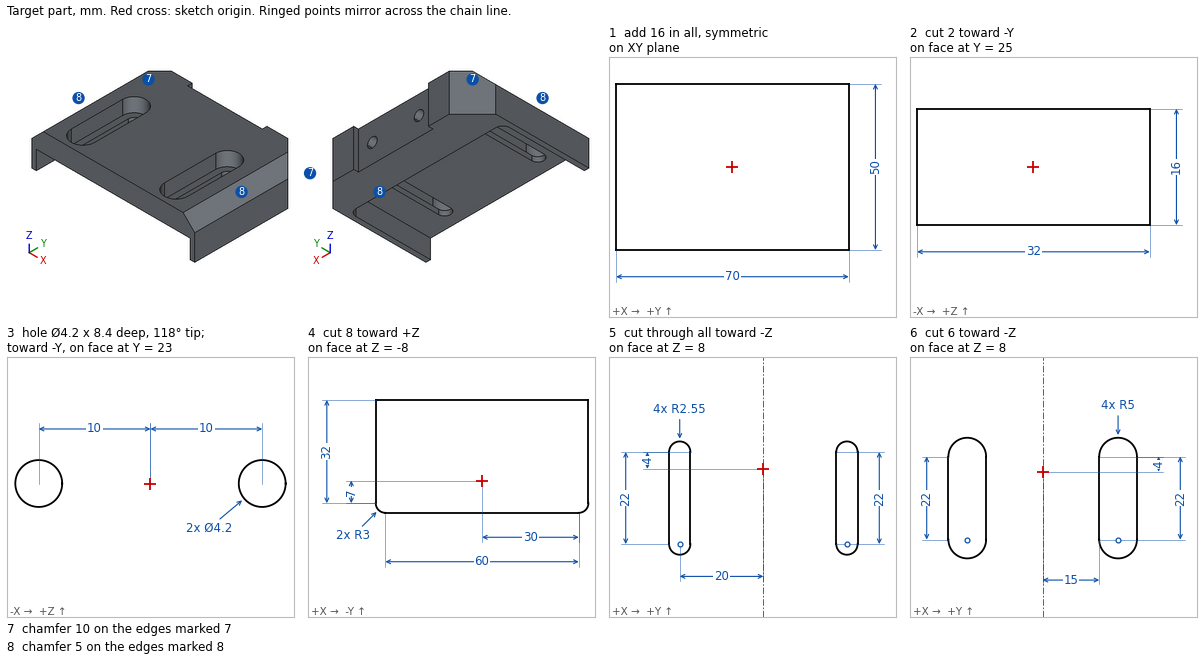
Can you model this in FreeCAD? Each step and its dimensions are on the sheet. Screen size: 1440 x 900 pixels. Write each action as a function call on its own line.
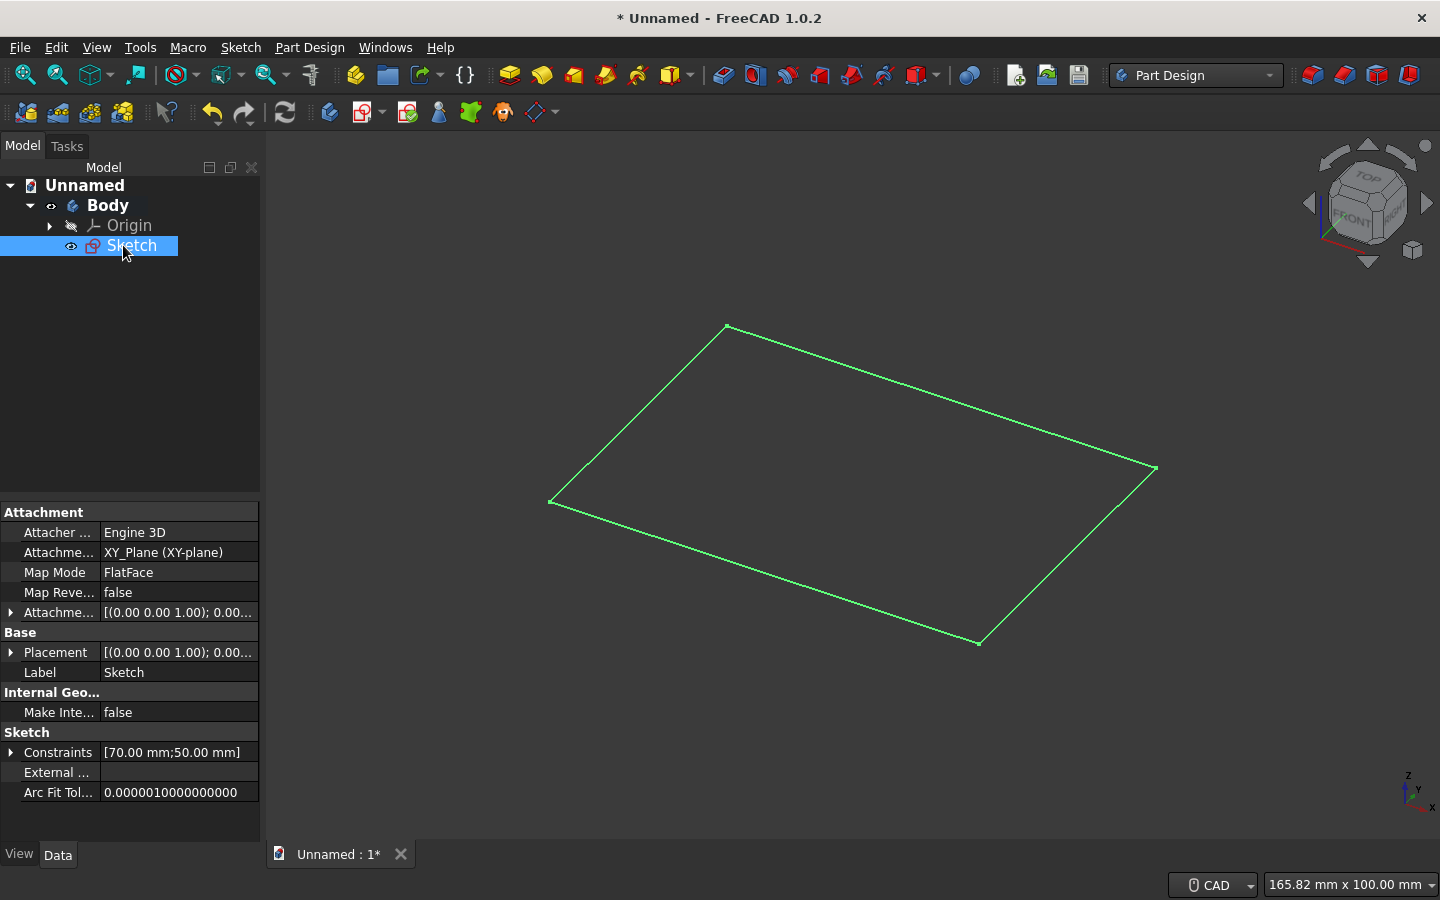
click(510, 76)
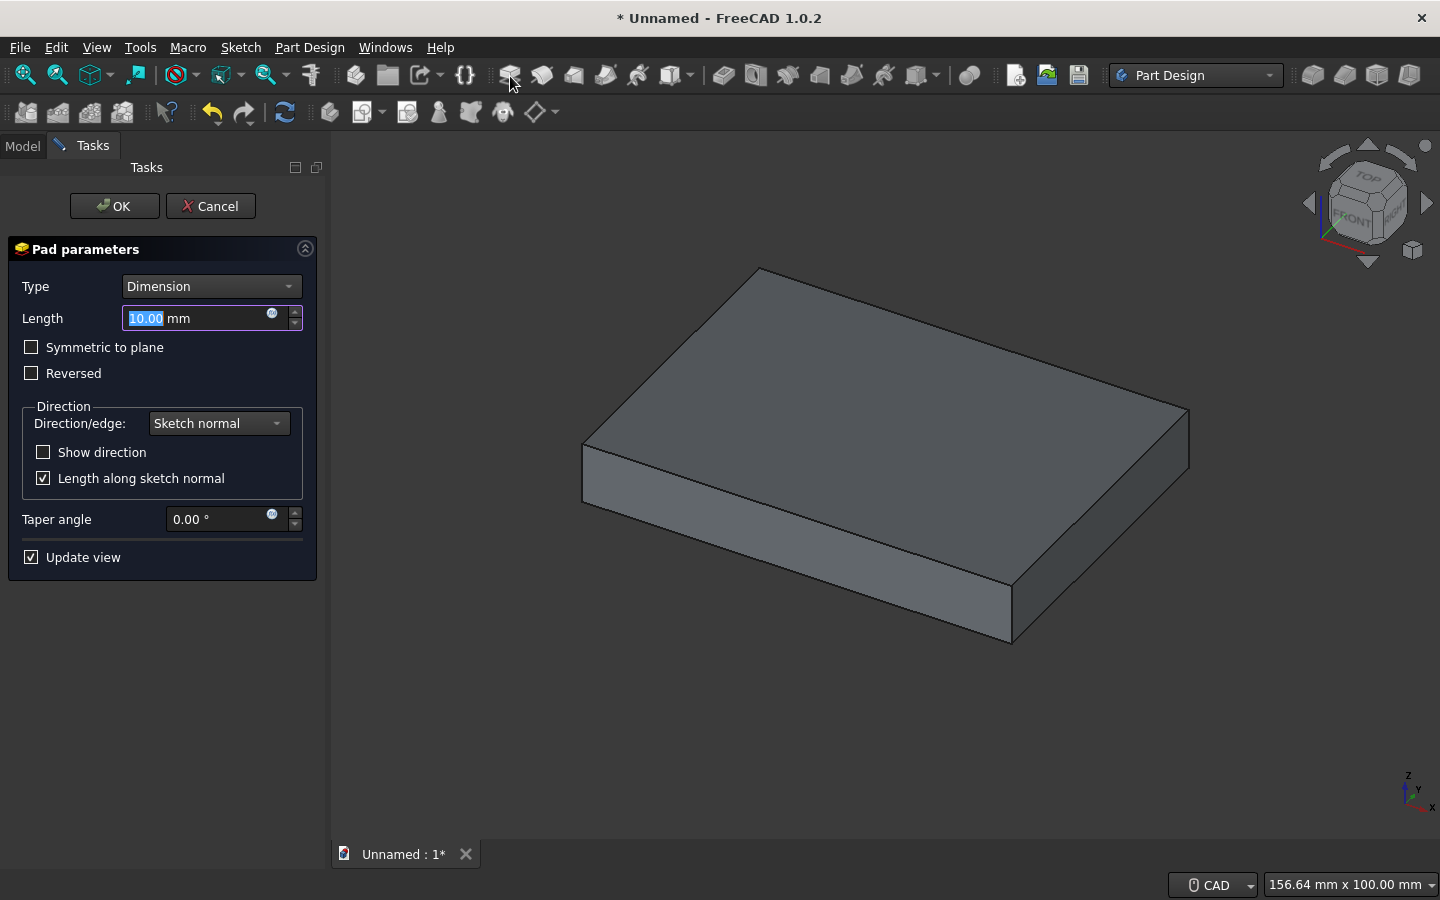
text(16)
key(Tab)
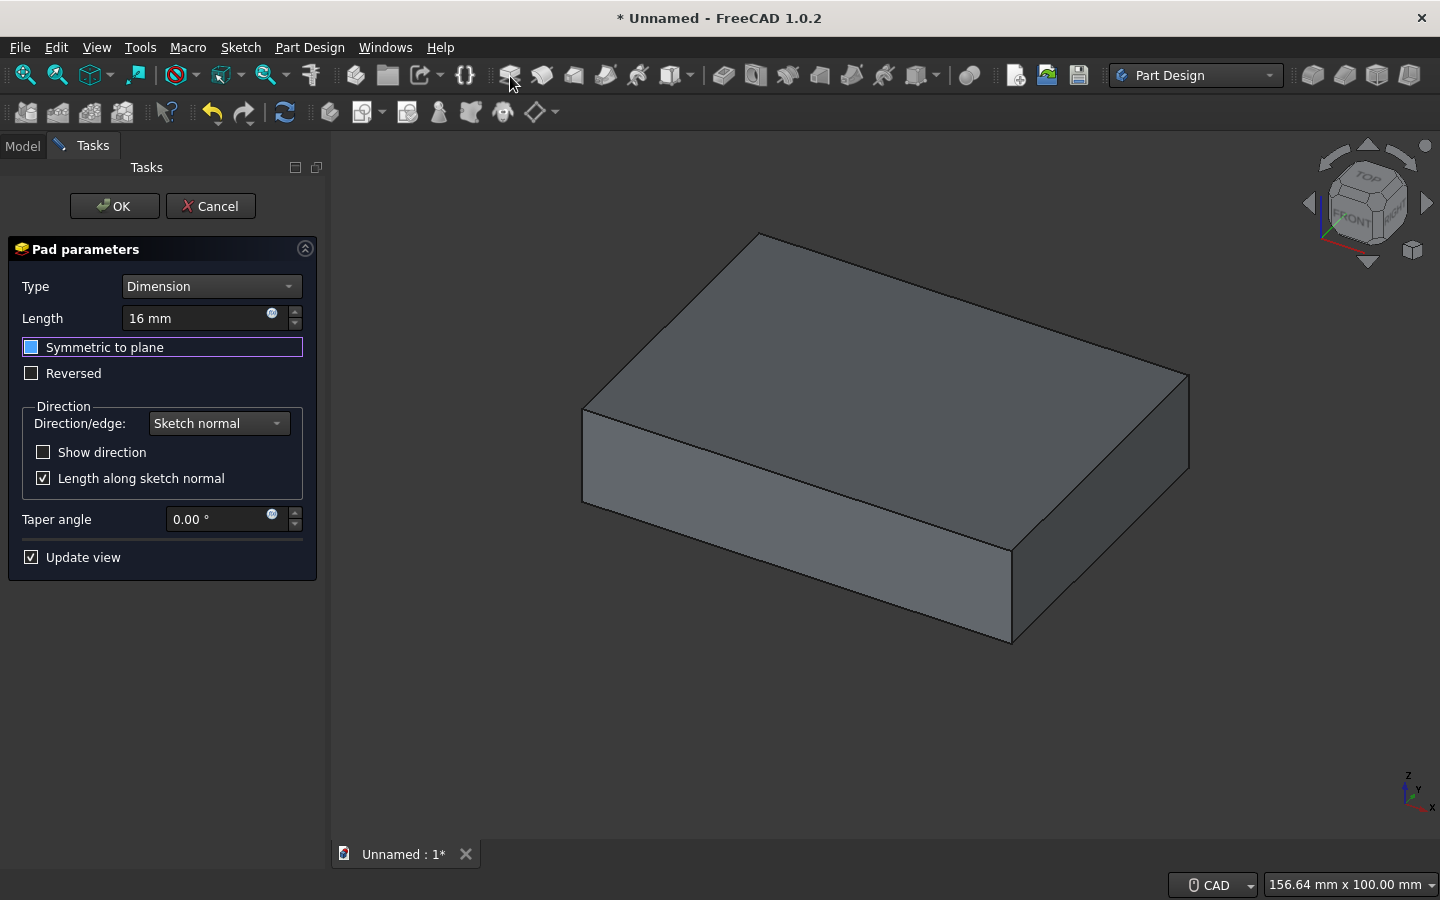
click(30, 347)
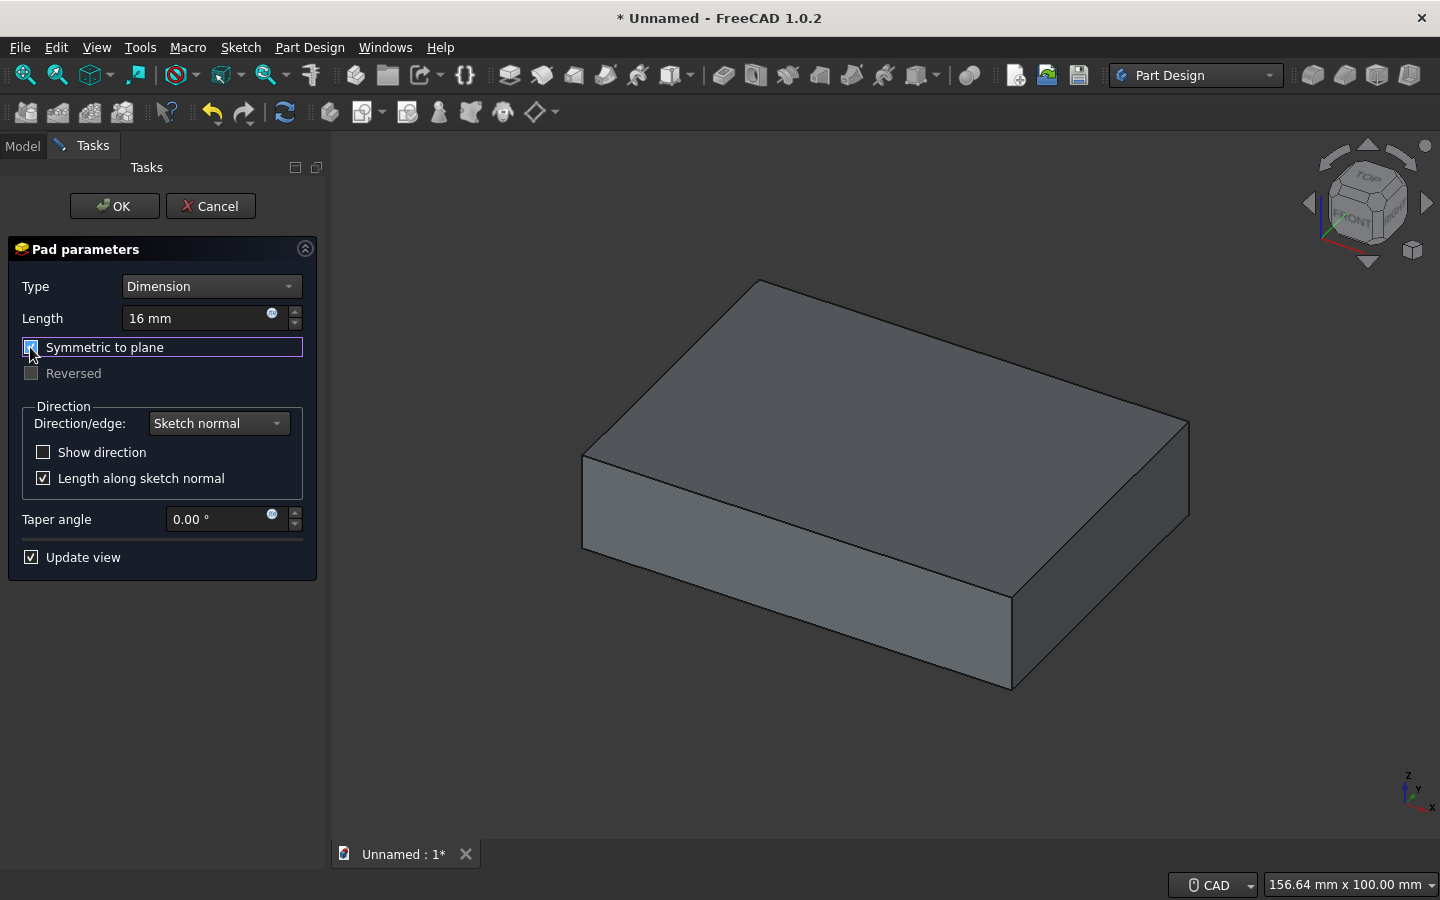
click(115, 206)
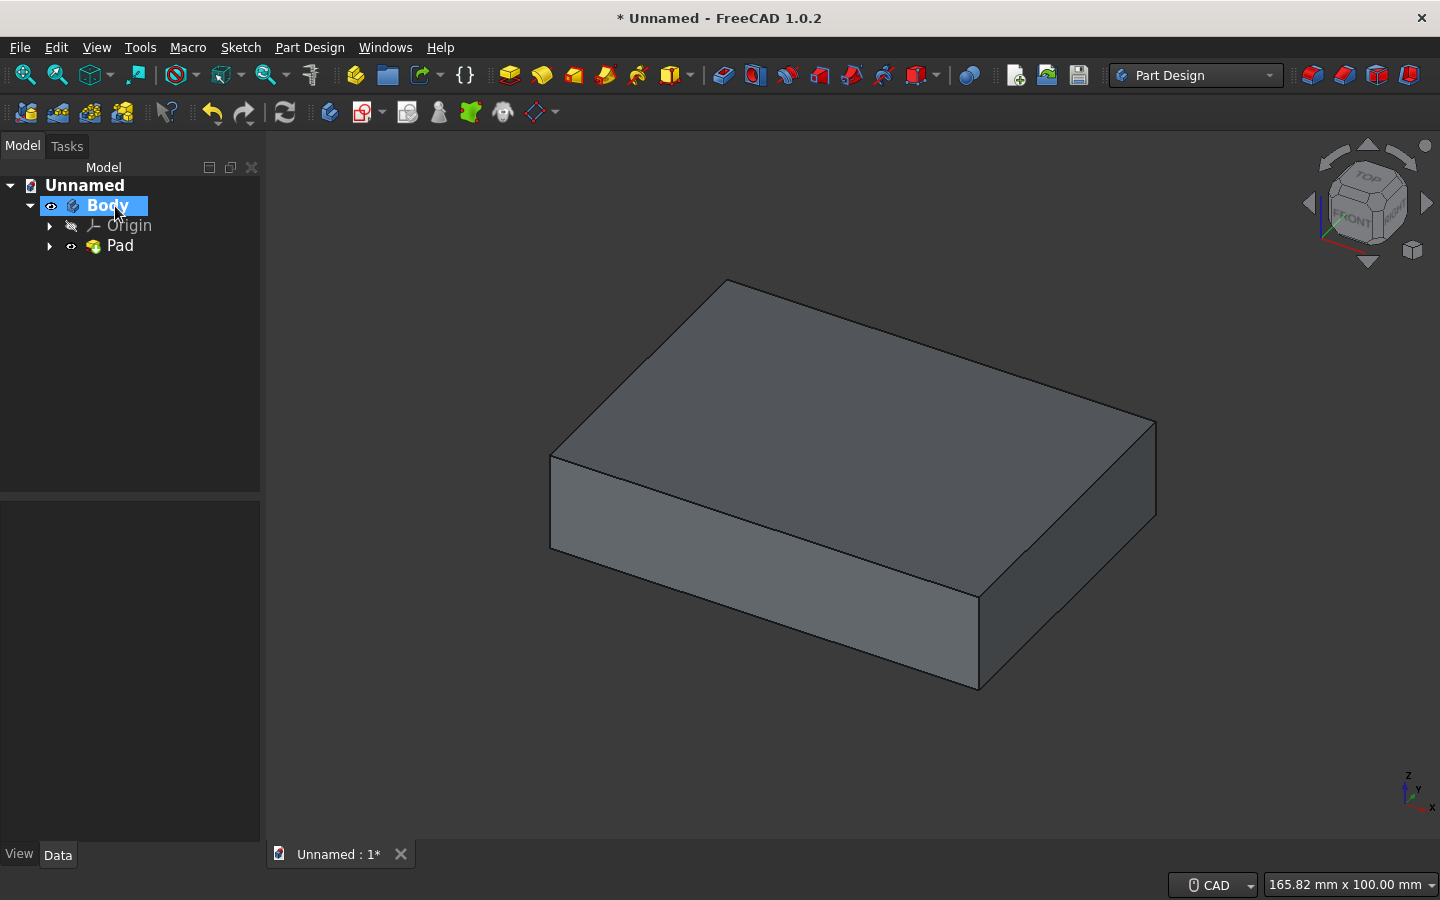
key(4)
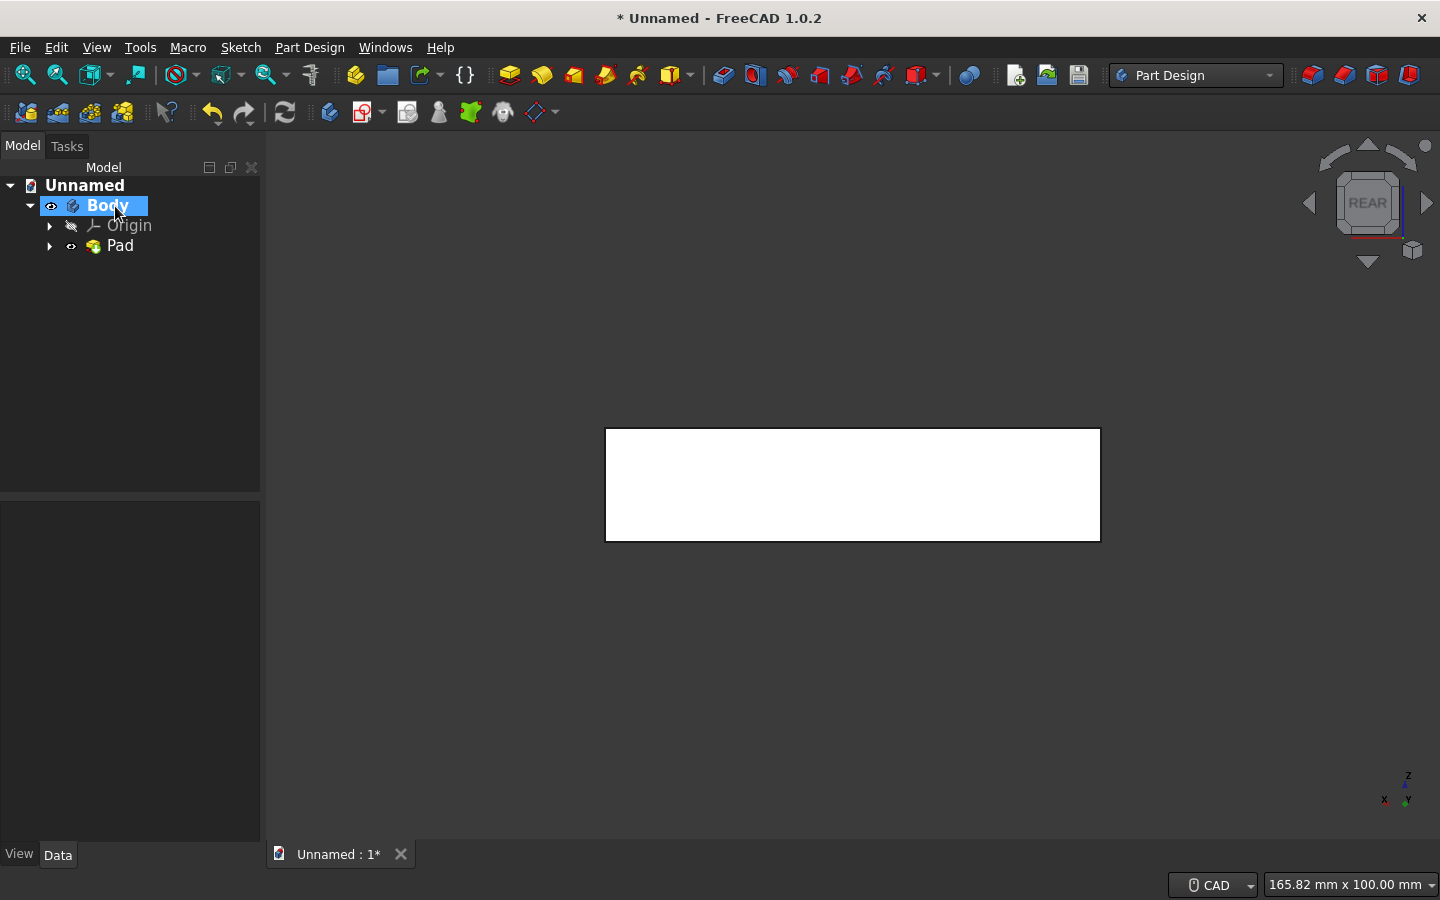
click(26, 76)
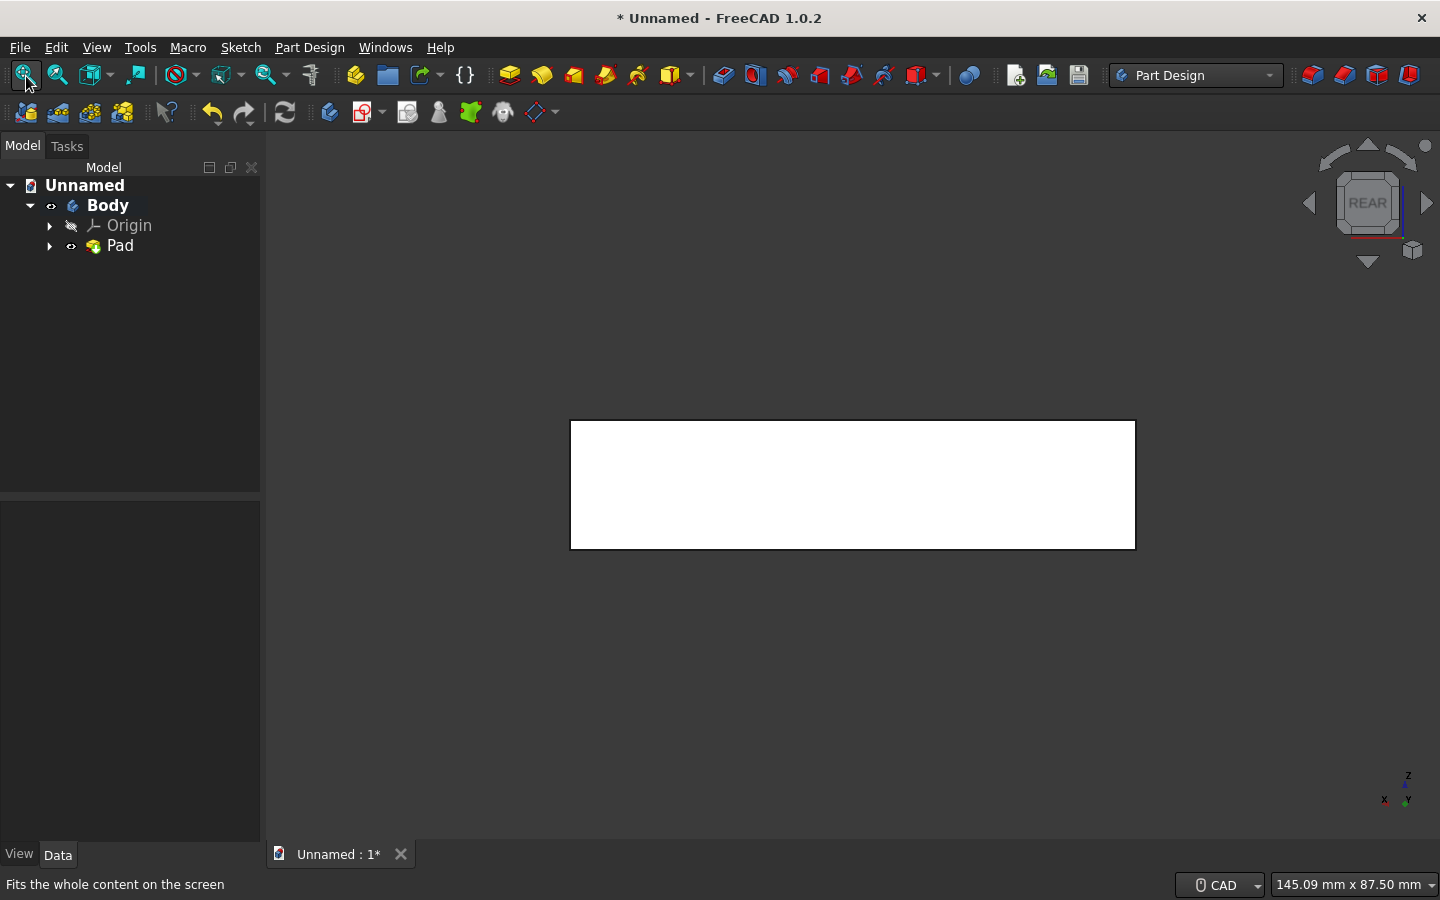
click(691, 484)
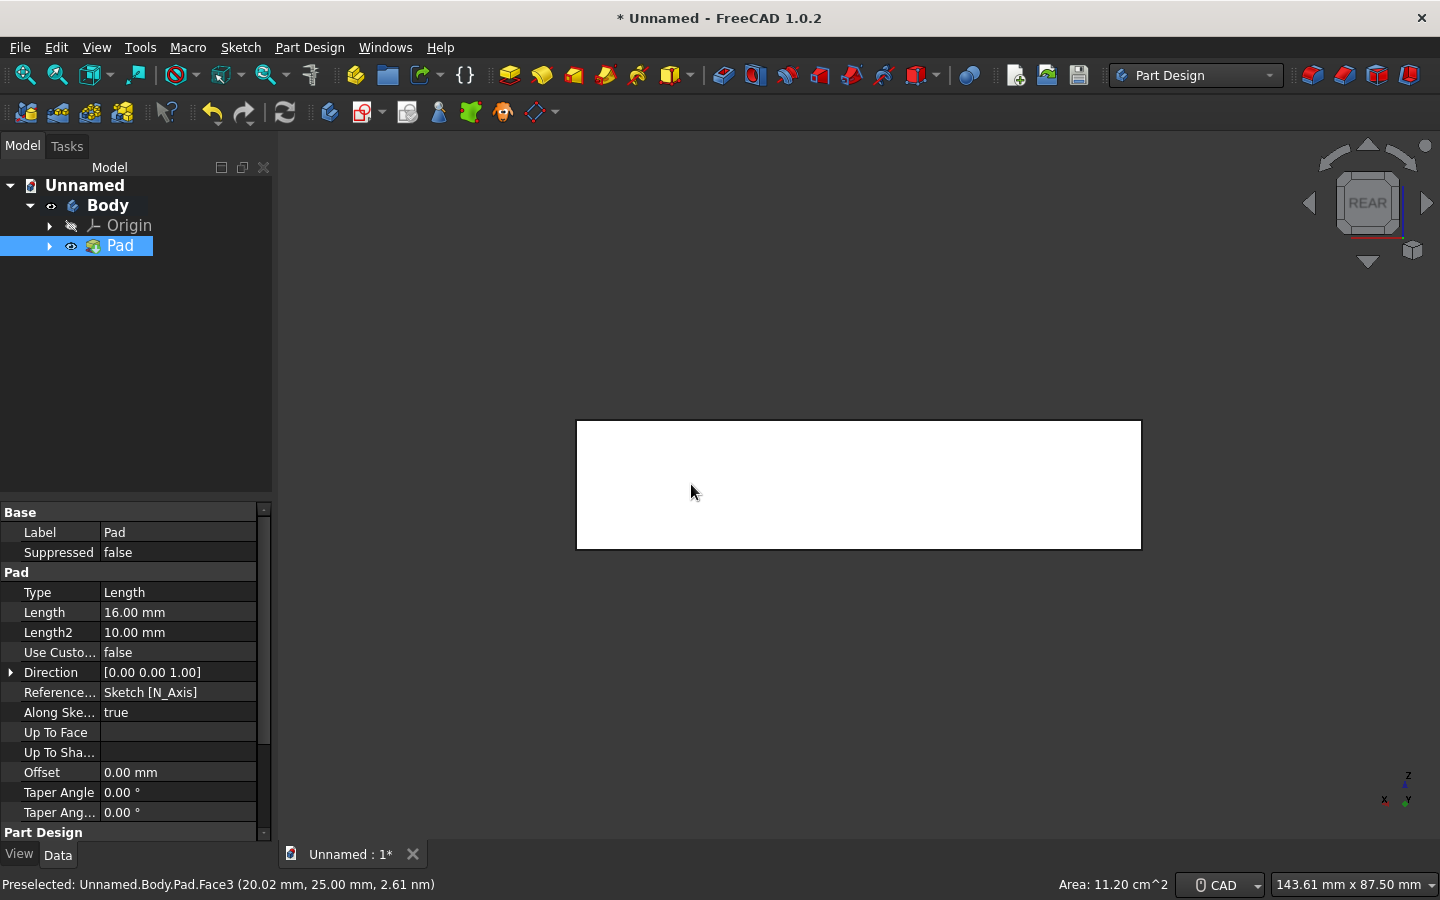
click(362, 112)